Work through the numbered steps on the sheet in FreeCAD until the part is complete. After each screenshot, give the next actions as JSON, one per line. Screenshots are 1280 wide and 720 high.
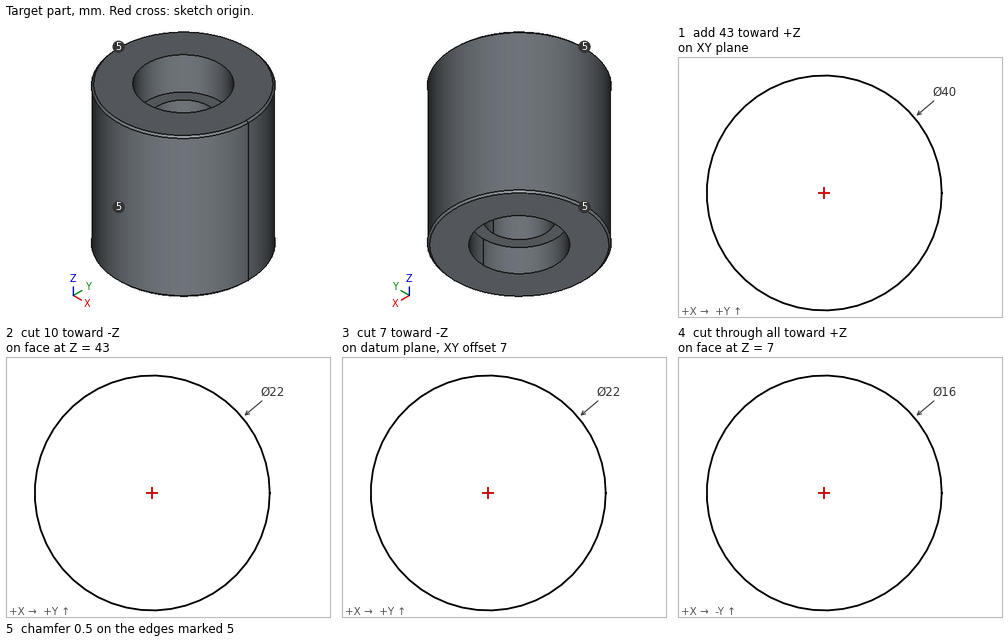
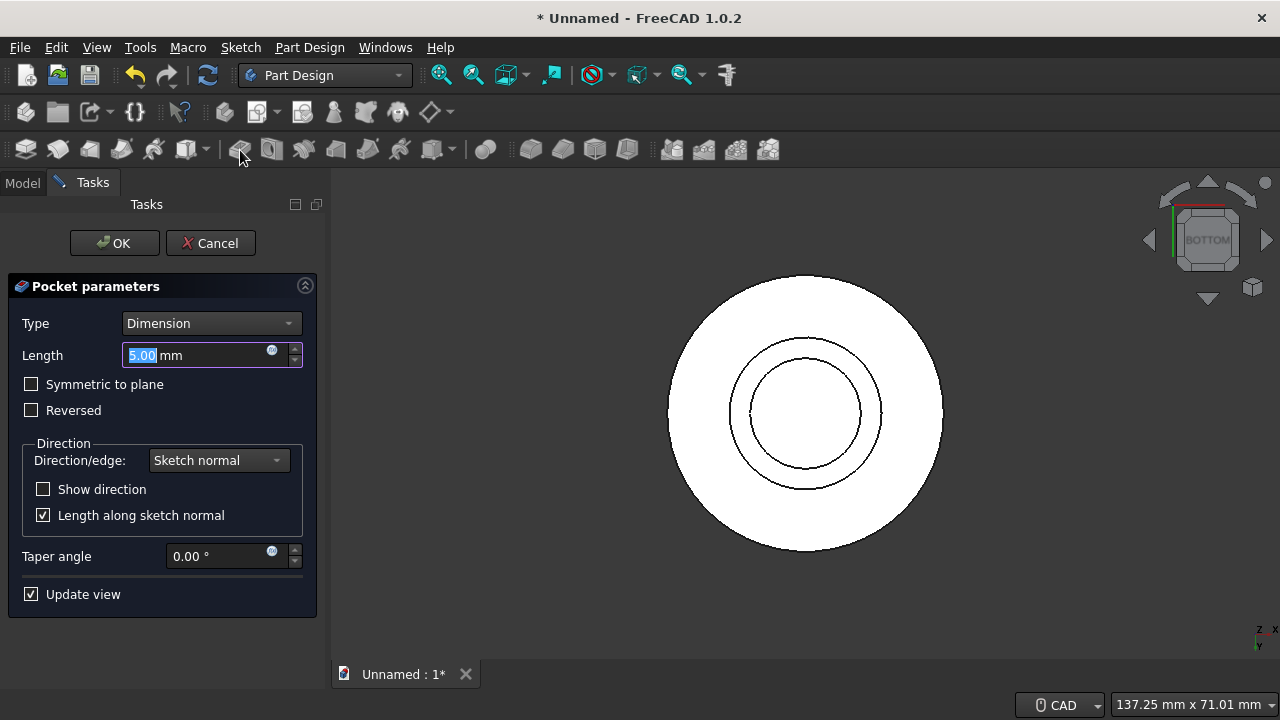
{"action": "left_click", "coordinate": [212, 324]}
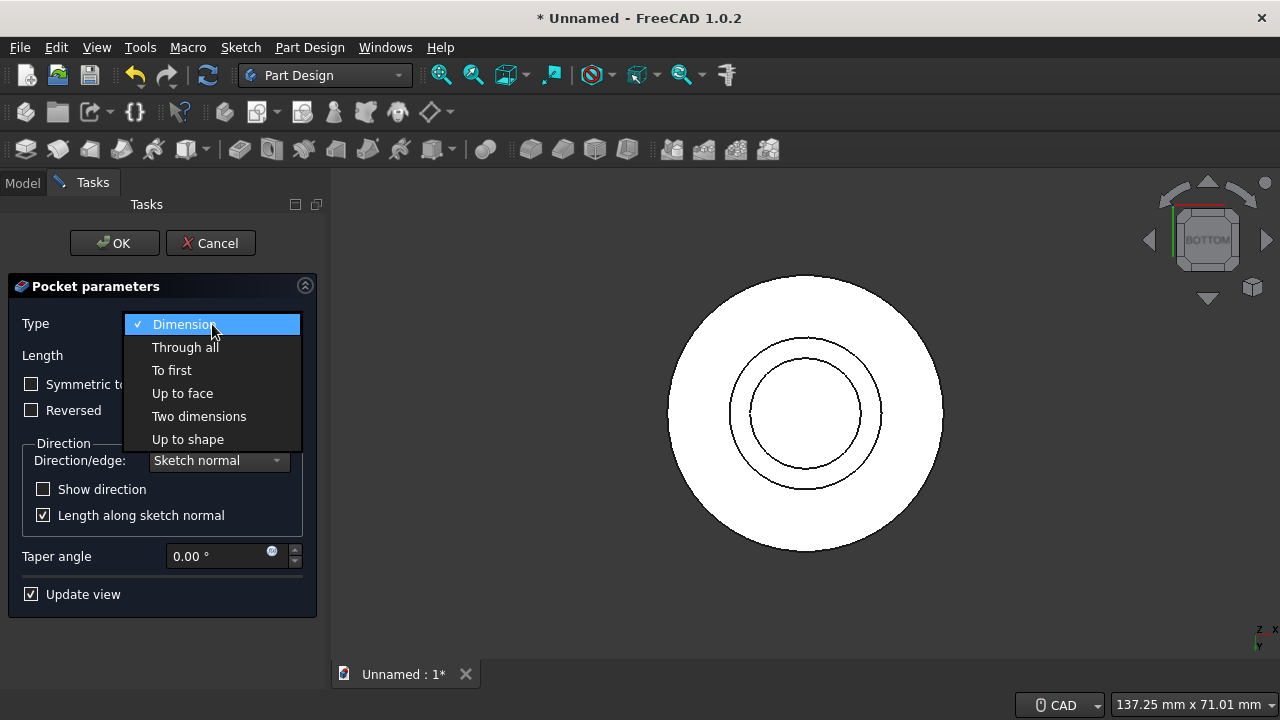
{"action": "left_click", "coordinate": [212, 348]}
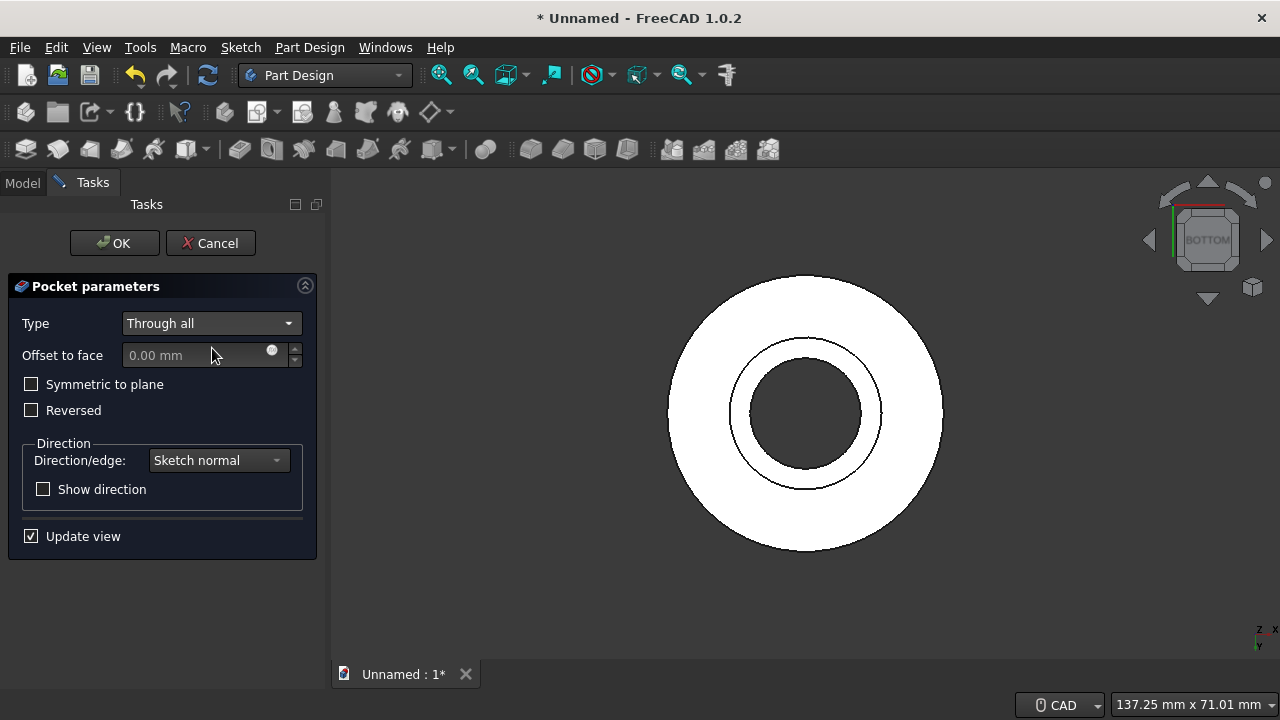
{"action": "left_click", "coordinate": [115, 243]}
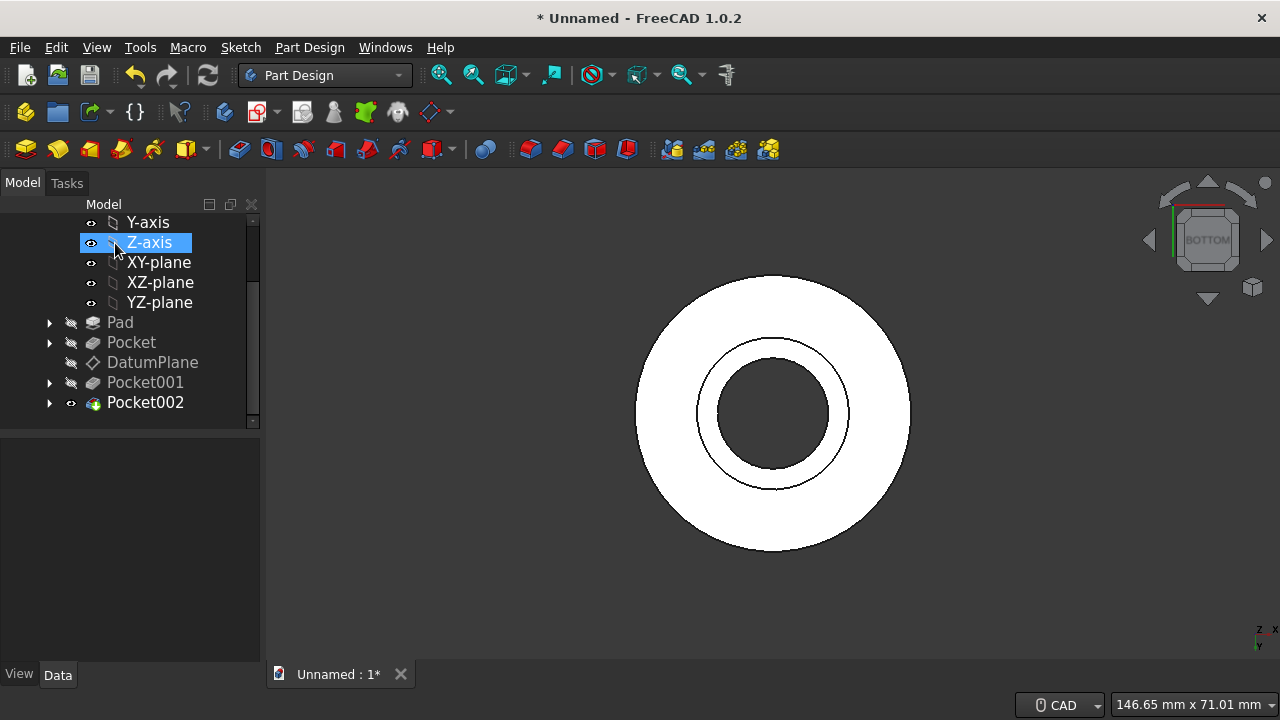
{"action": "left_click", "coordinate": [635, 412]}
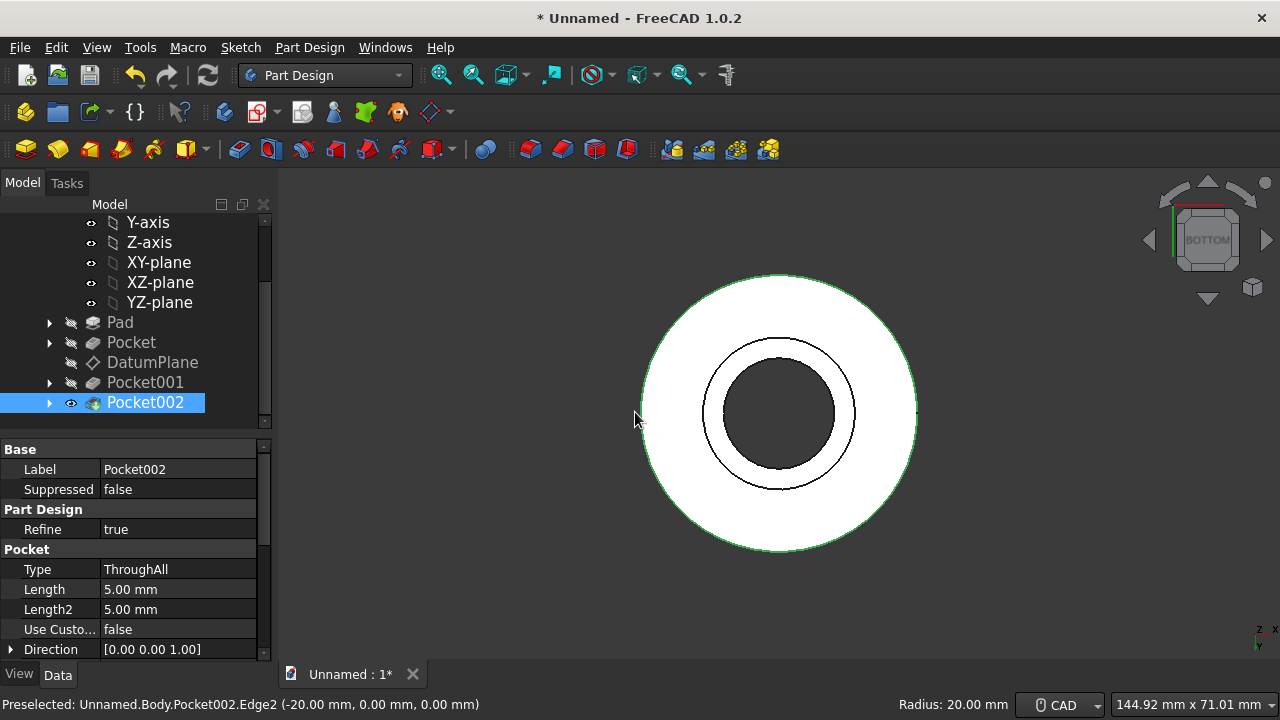
{"action": "key", "text": "0"}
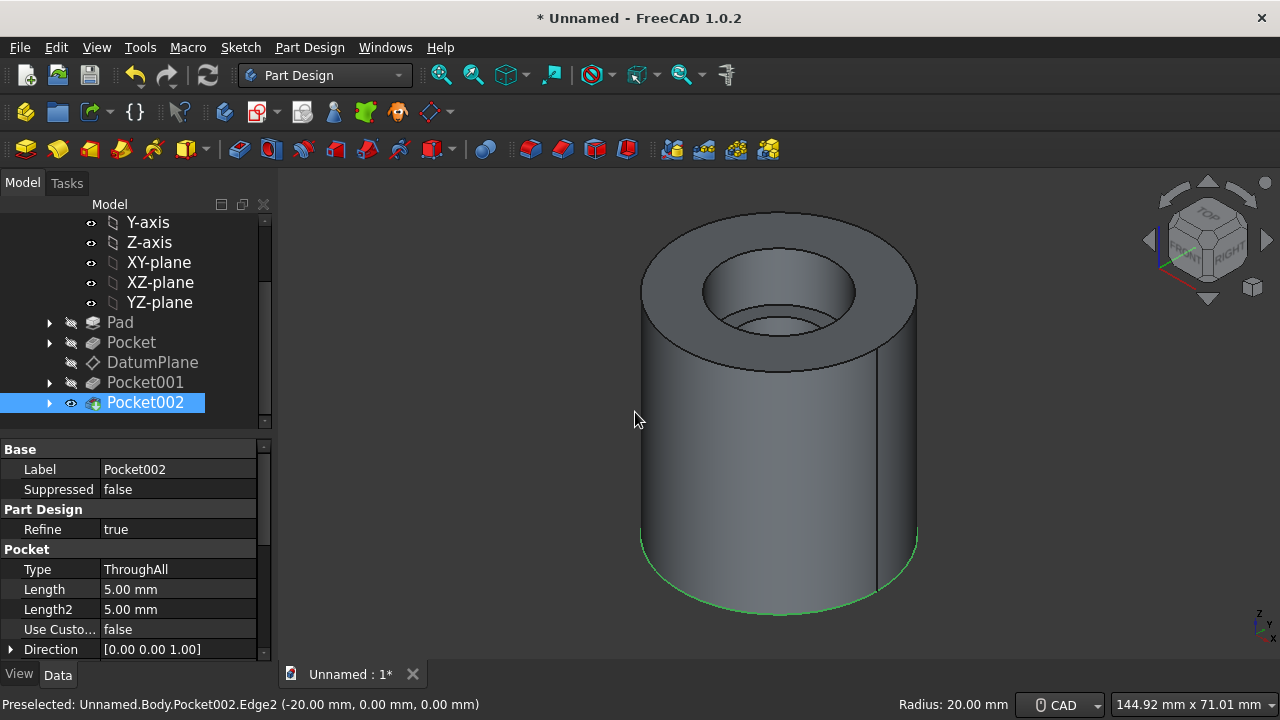
{"action": "left_click", "coordinate": [656, 327], "text": "ctrl"}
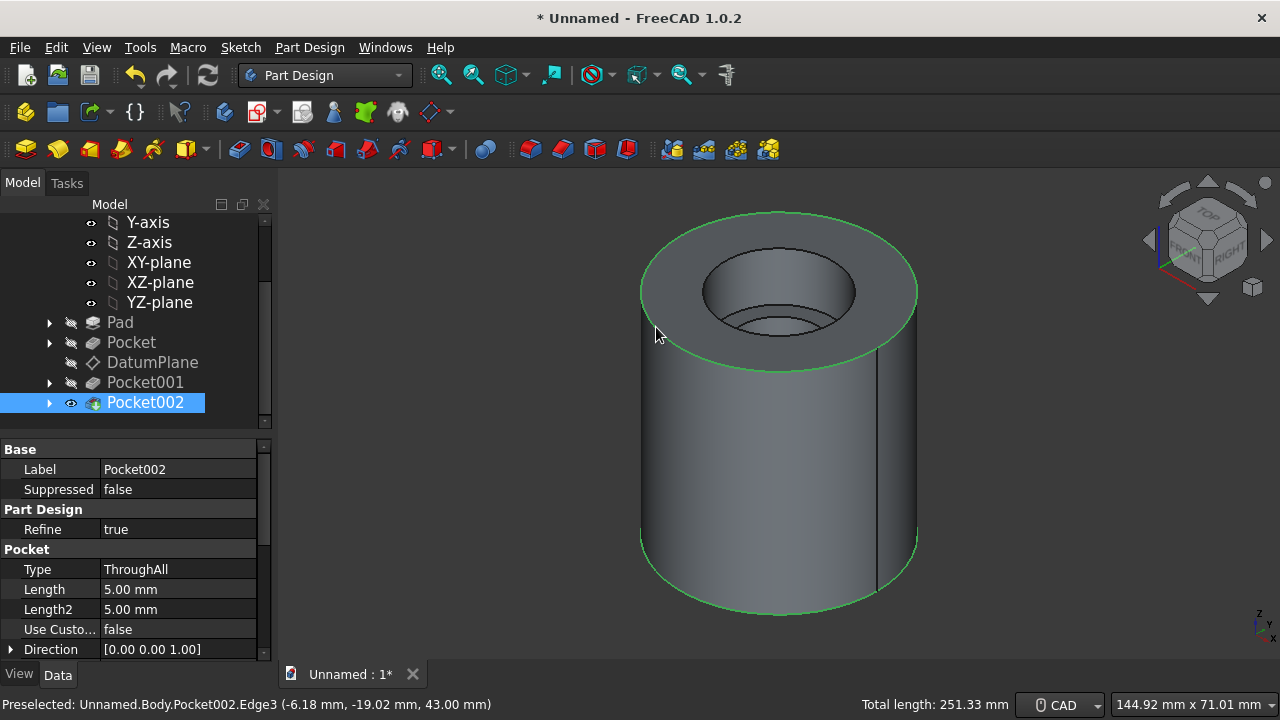
{"action": "left_click", "coordinate": [564, 150]}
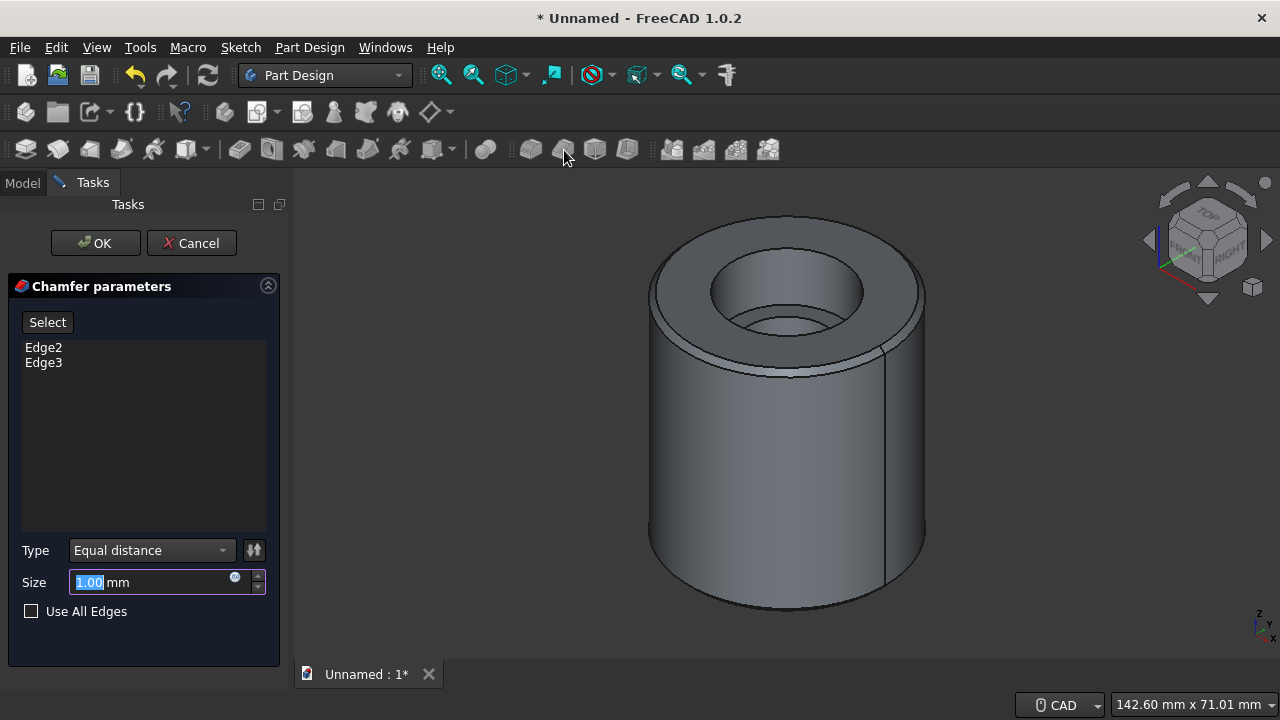
{"action": "type", "text": "0.5"}
{"action": "key", "text": "Tab"}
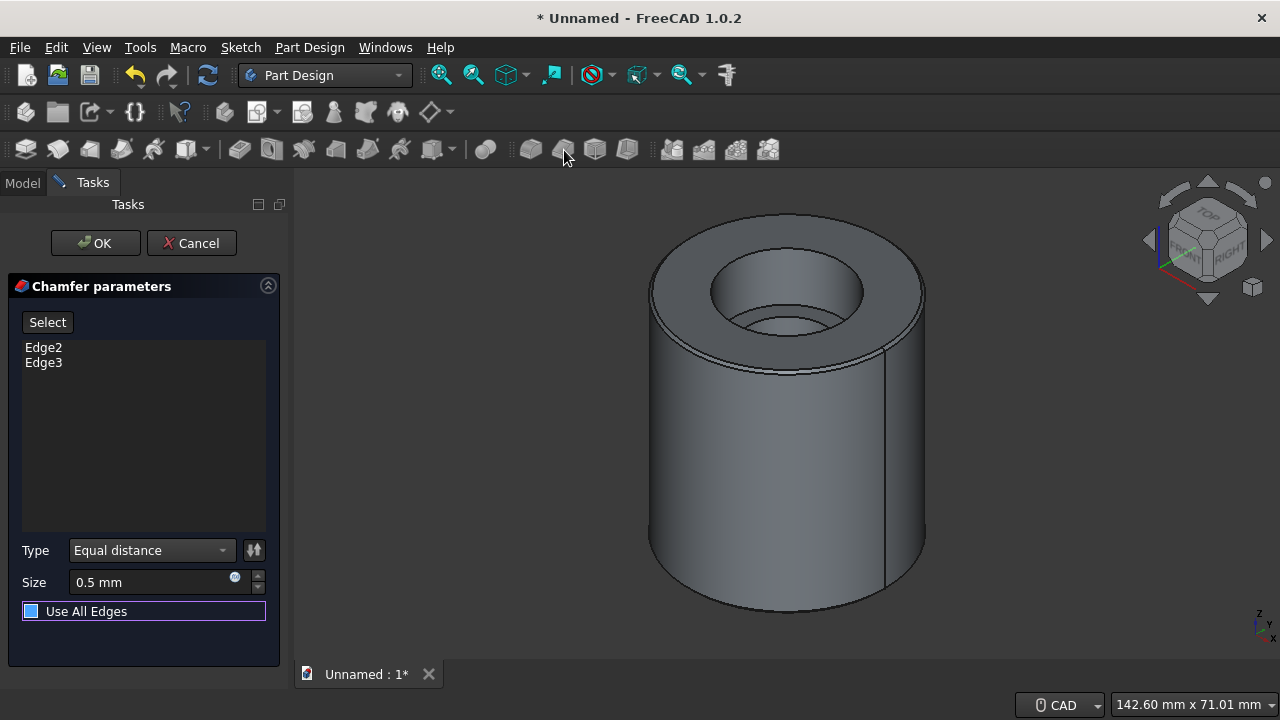
{"action": "left_click", "coordinate": [96, 243]}